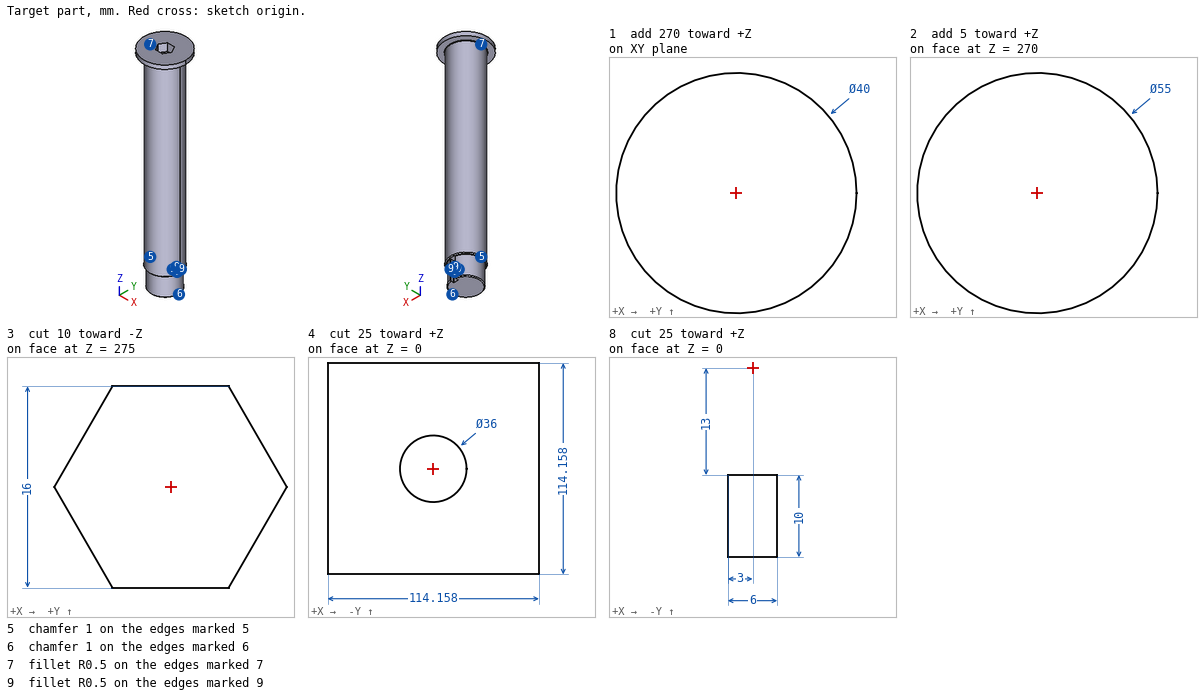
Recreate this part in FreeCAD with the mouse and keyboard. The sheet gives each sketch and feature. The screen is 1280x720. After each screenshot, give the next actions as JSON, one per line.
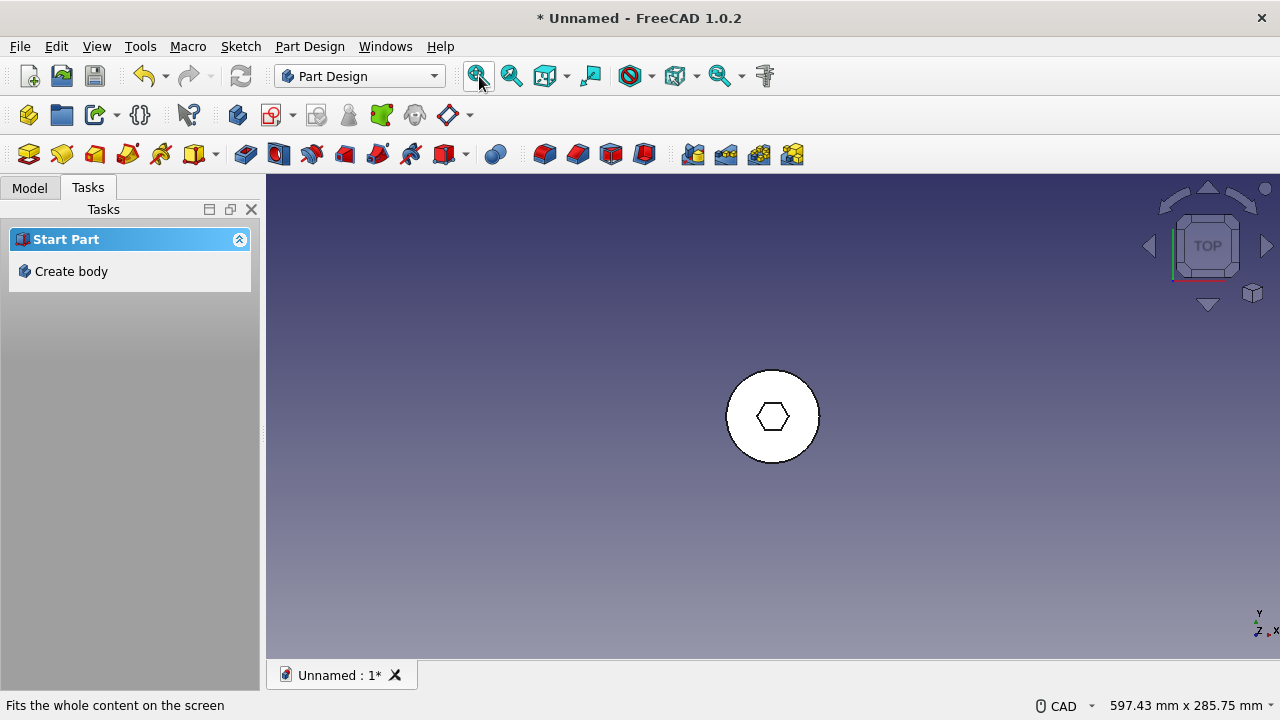
{"action": "left_click", "coordinate": [479, 76]}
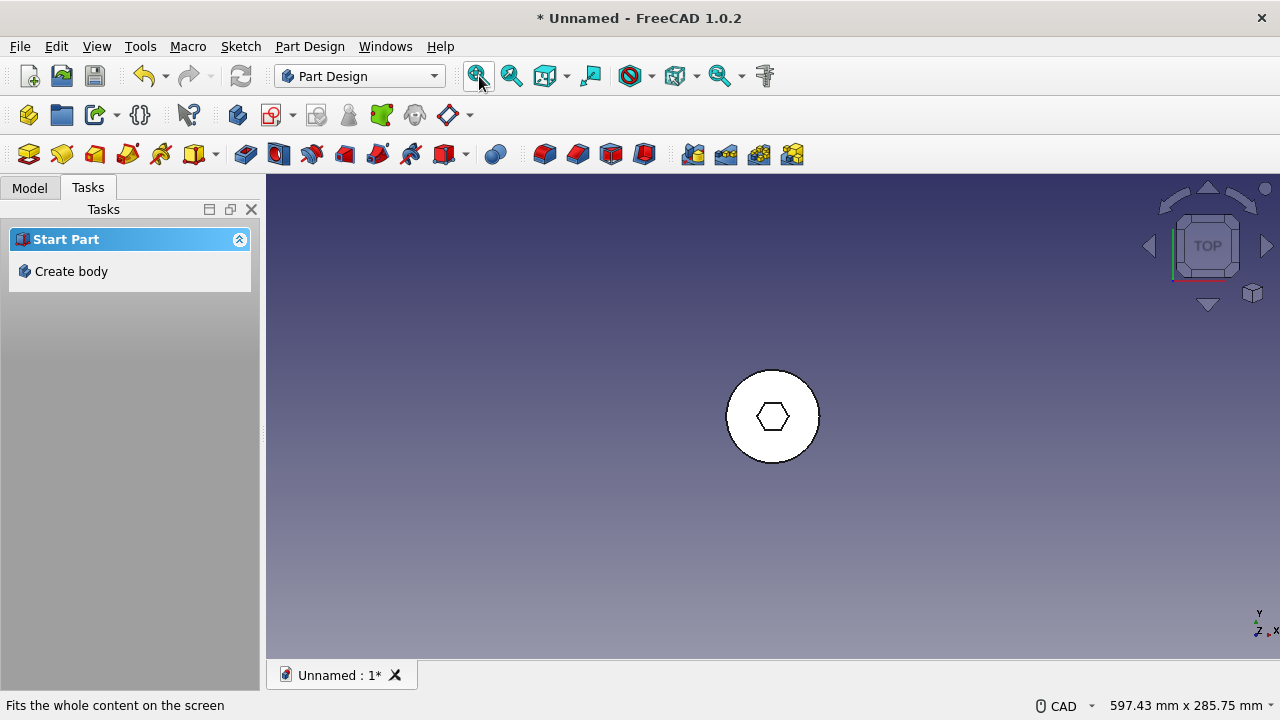
{"action": "key", "text": "1"}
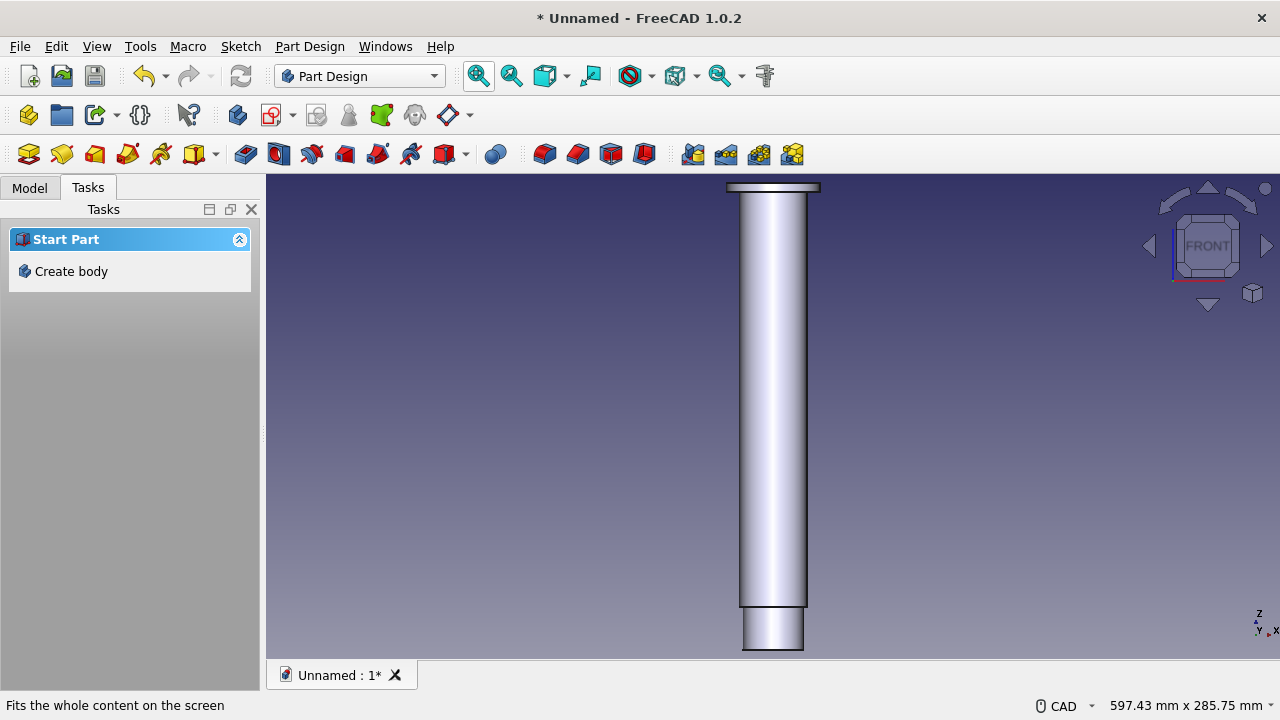
{"action": "left_click", "coordinate": [745, 606]}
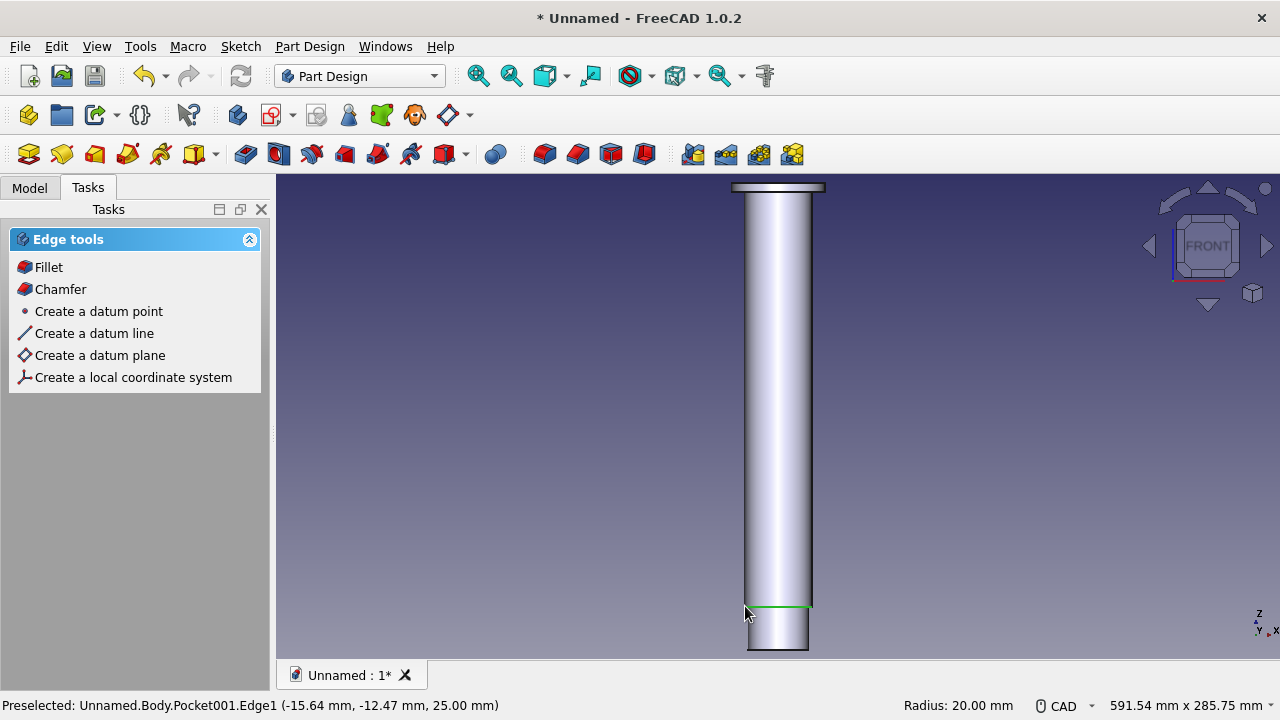
{"action": "left_click", "coordinate": [578, 154]}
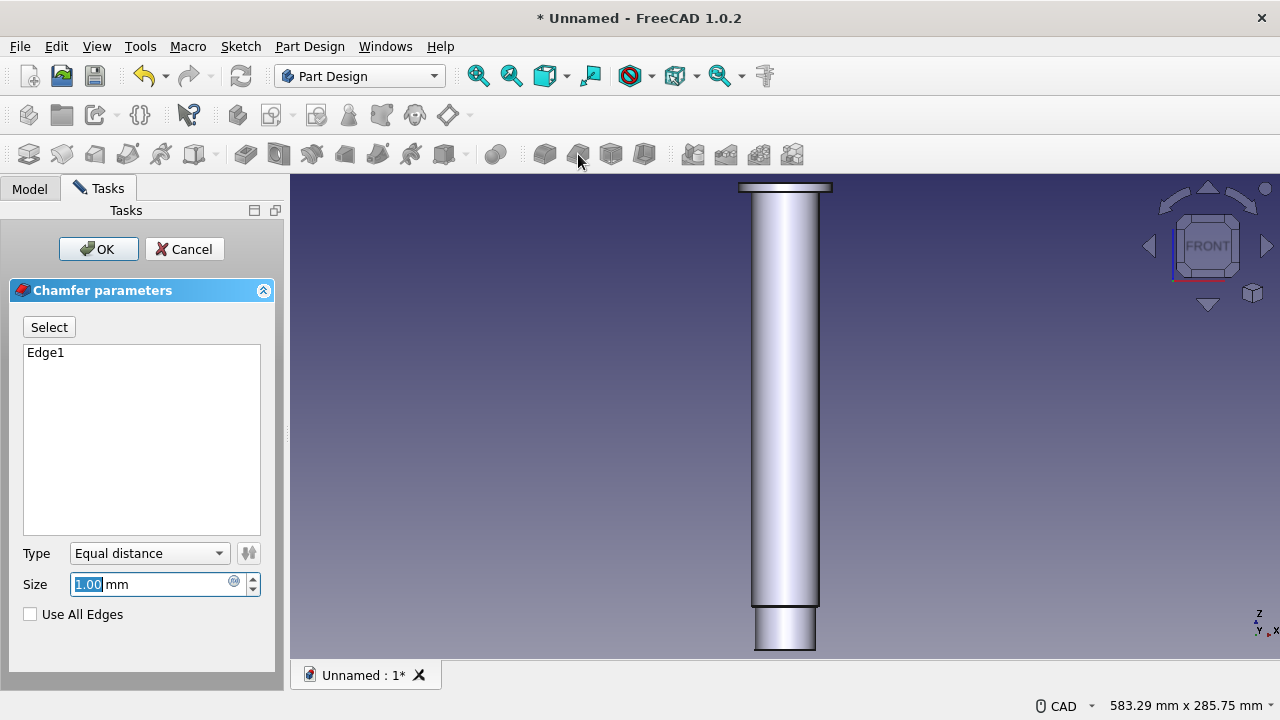
{"action": "type", "text": "1"}
{"action": "key", "text": "Tab"}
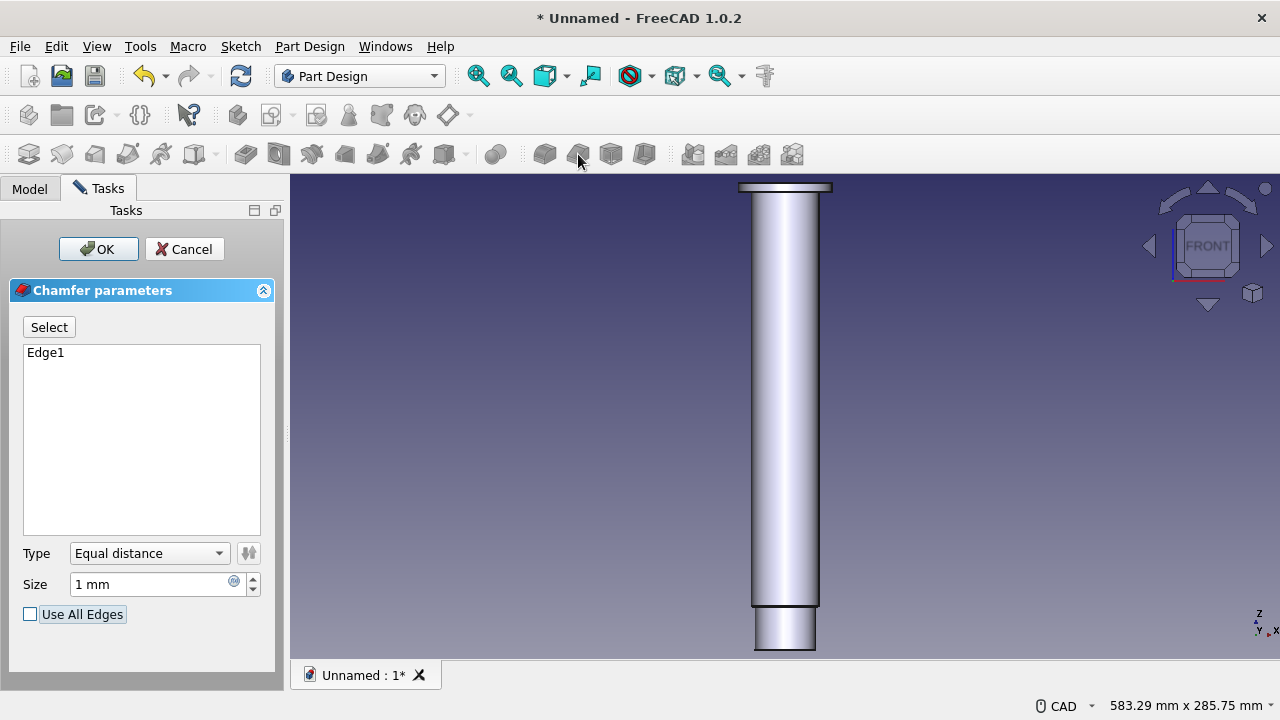
{"action": "left_click", "coordinate": [99, 249]}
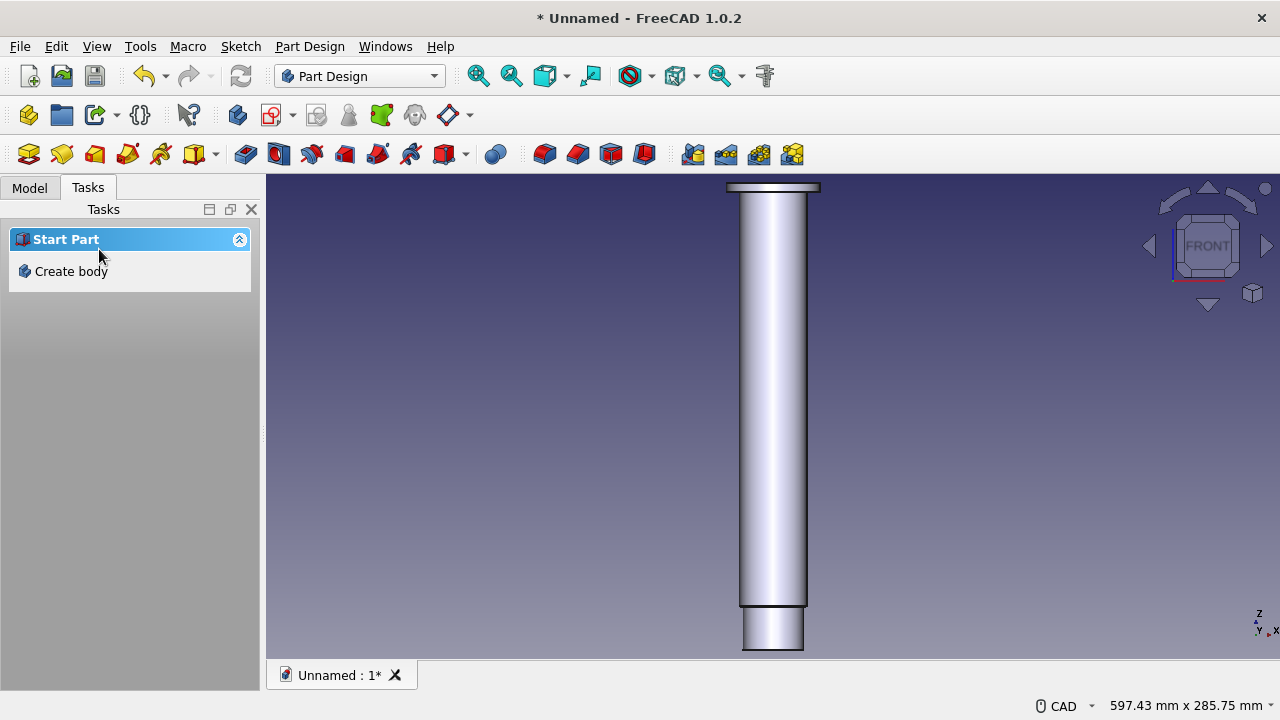
{"action": "key", "text": "0"}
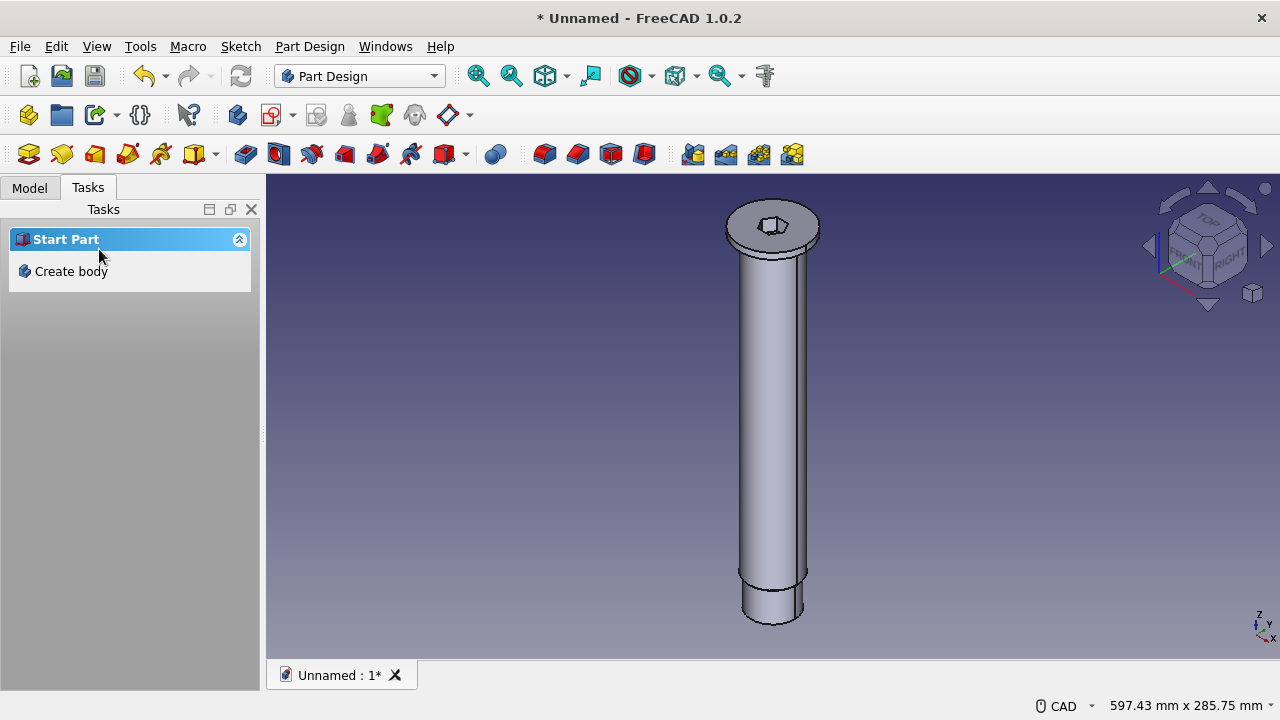
{"action": "left_click", "coordinate": [759, 622]}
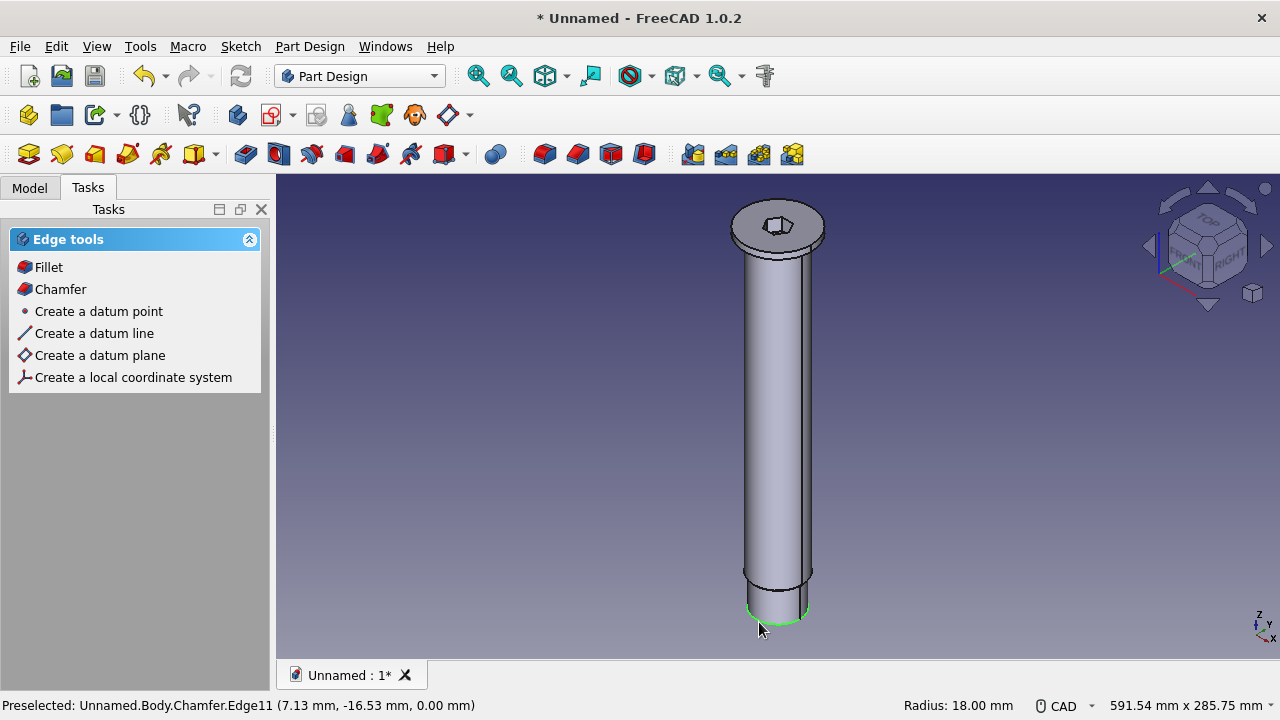
{"action": "left_click", "coordinate": [578, 154]}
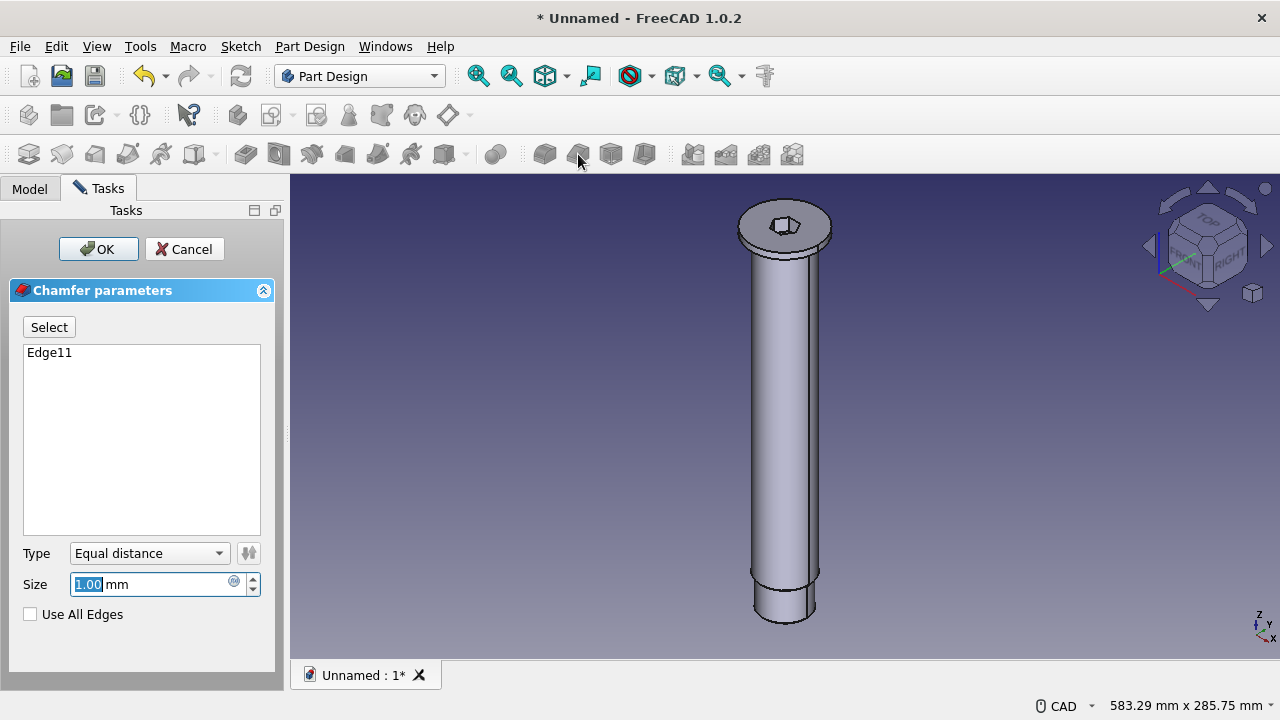
{"action": "type", "text": "1"}
{"action": "key", "text": "Tab"}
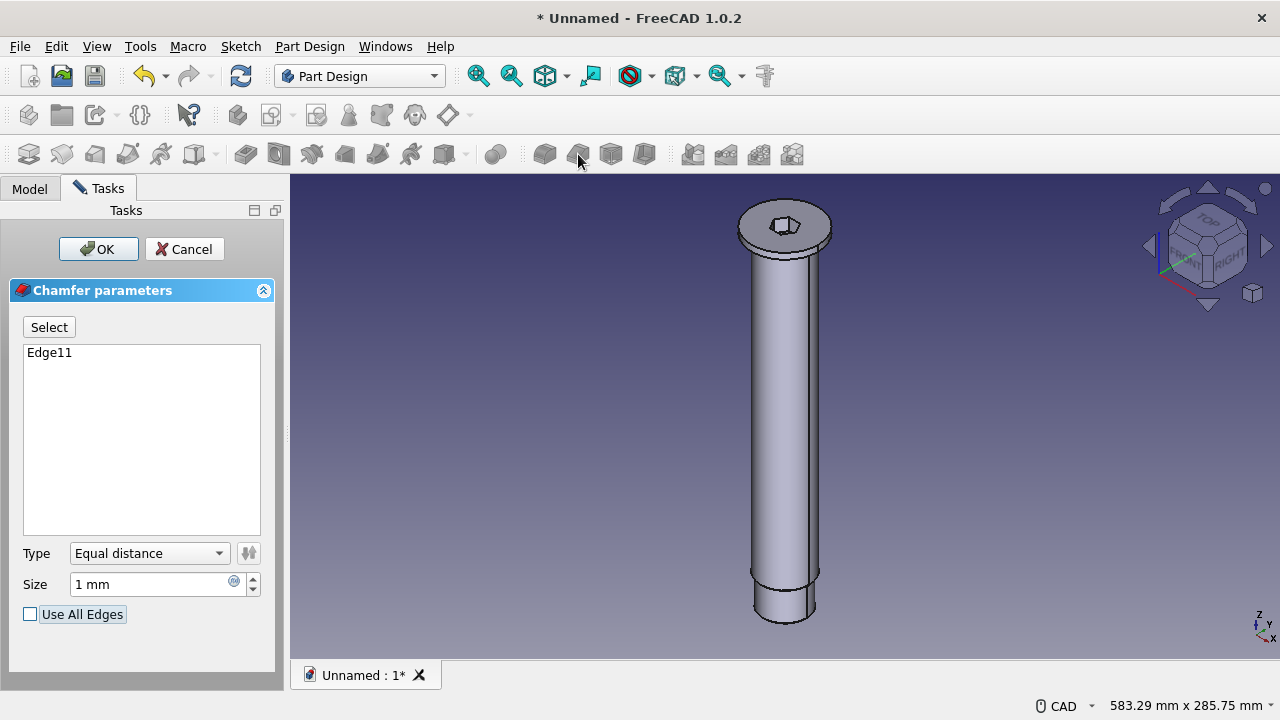
{"action": "left_click", "coordinate": [99, 249]}